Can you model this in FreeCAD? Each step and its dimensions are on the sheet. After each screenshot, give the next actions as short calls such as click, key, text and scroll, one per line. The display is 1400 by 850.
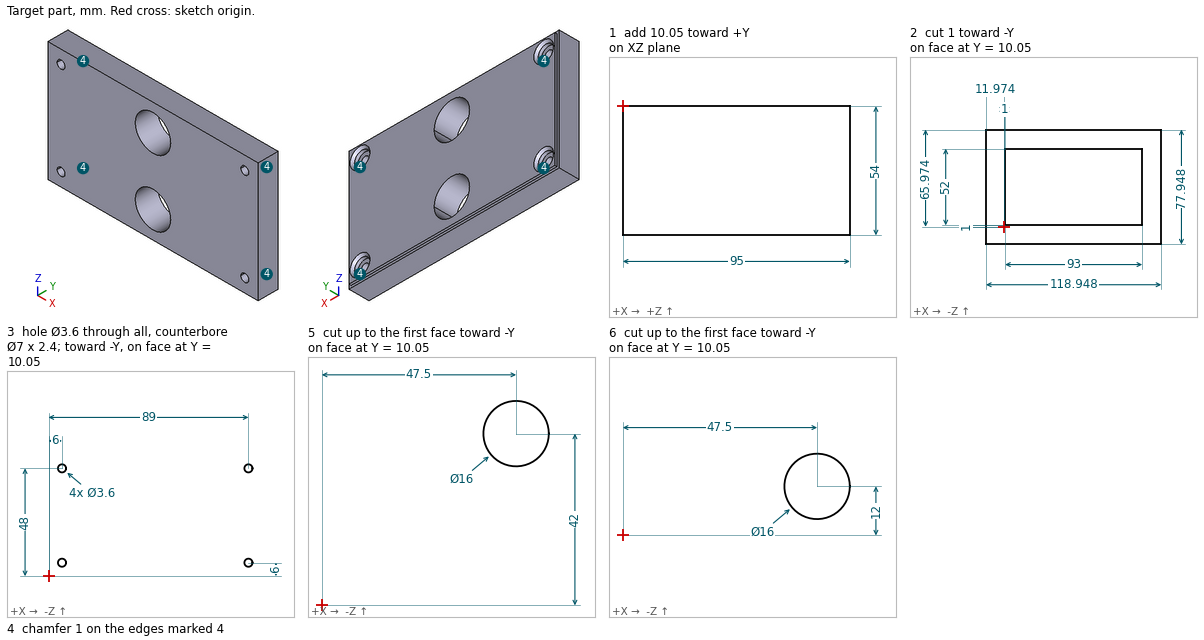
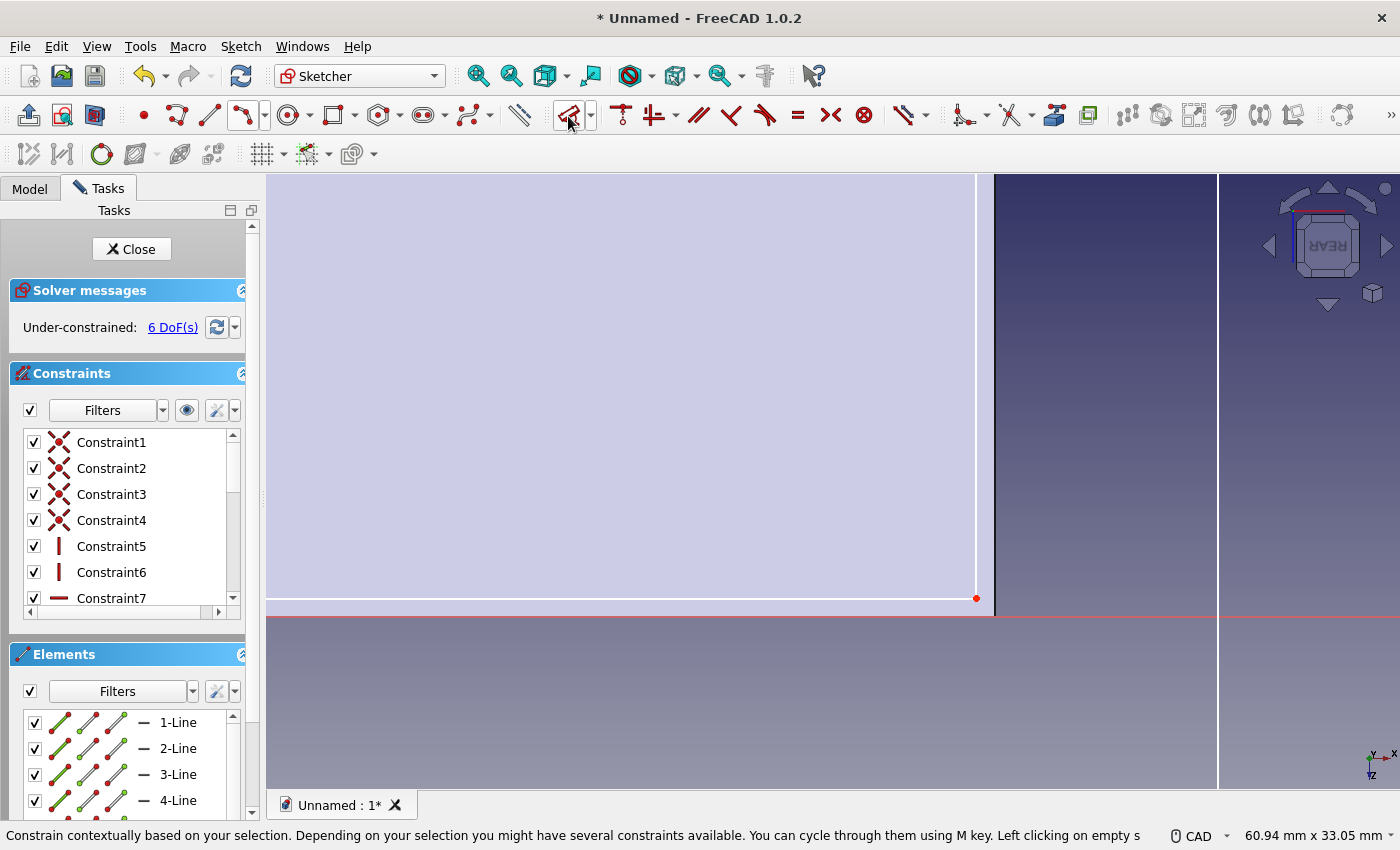
scroll(978, 602, down, 7)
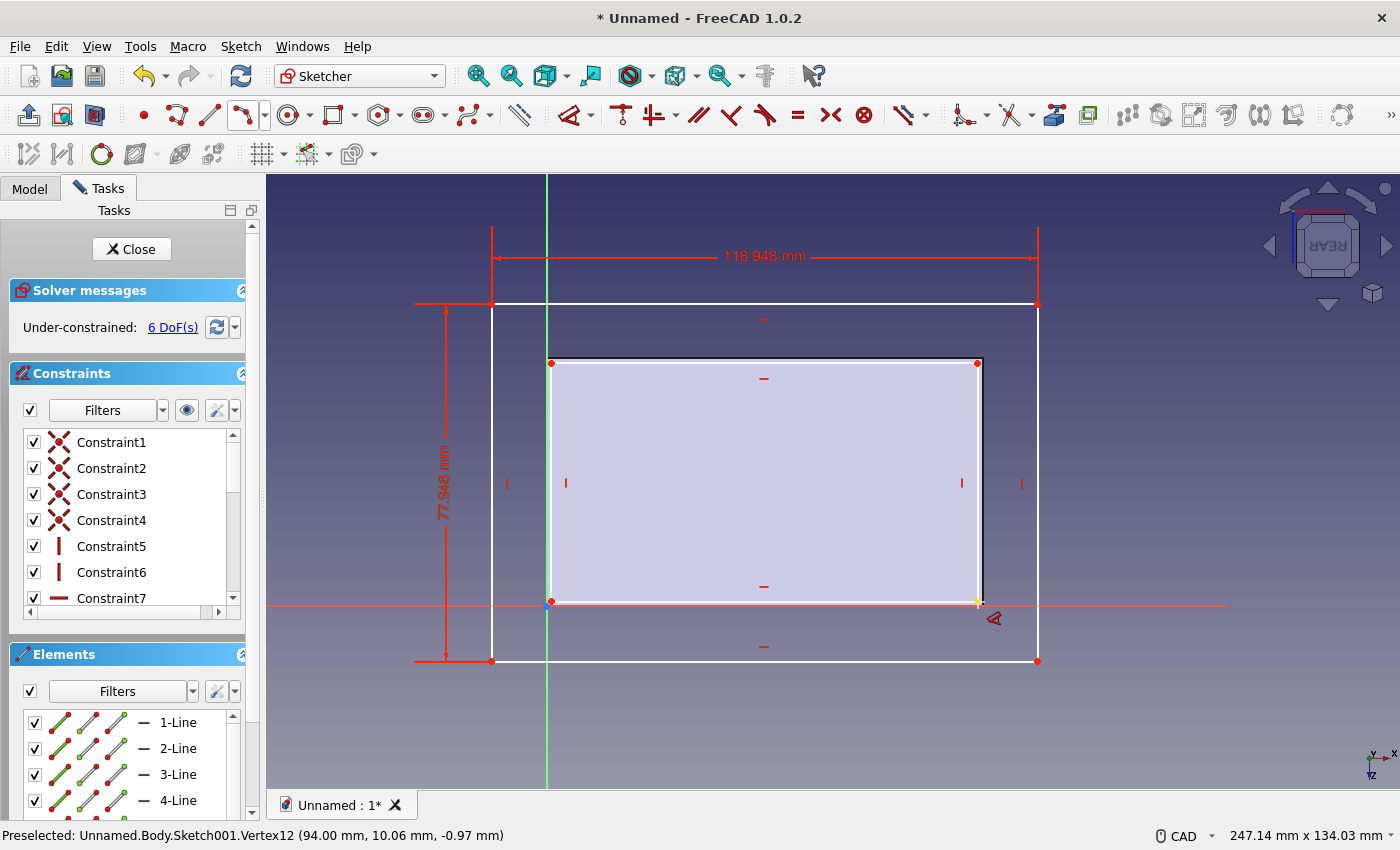
scroll(551, 435, up, 6)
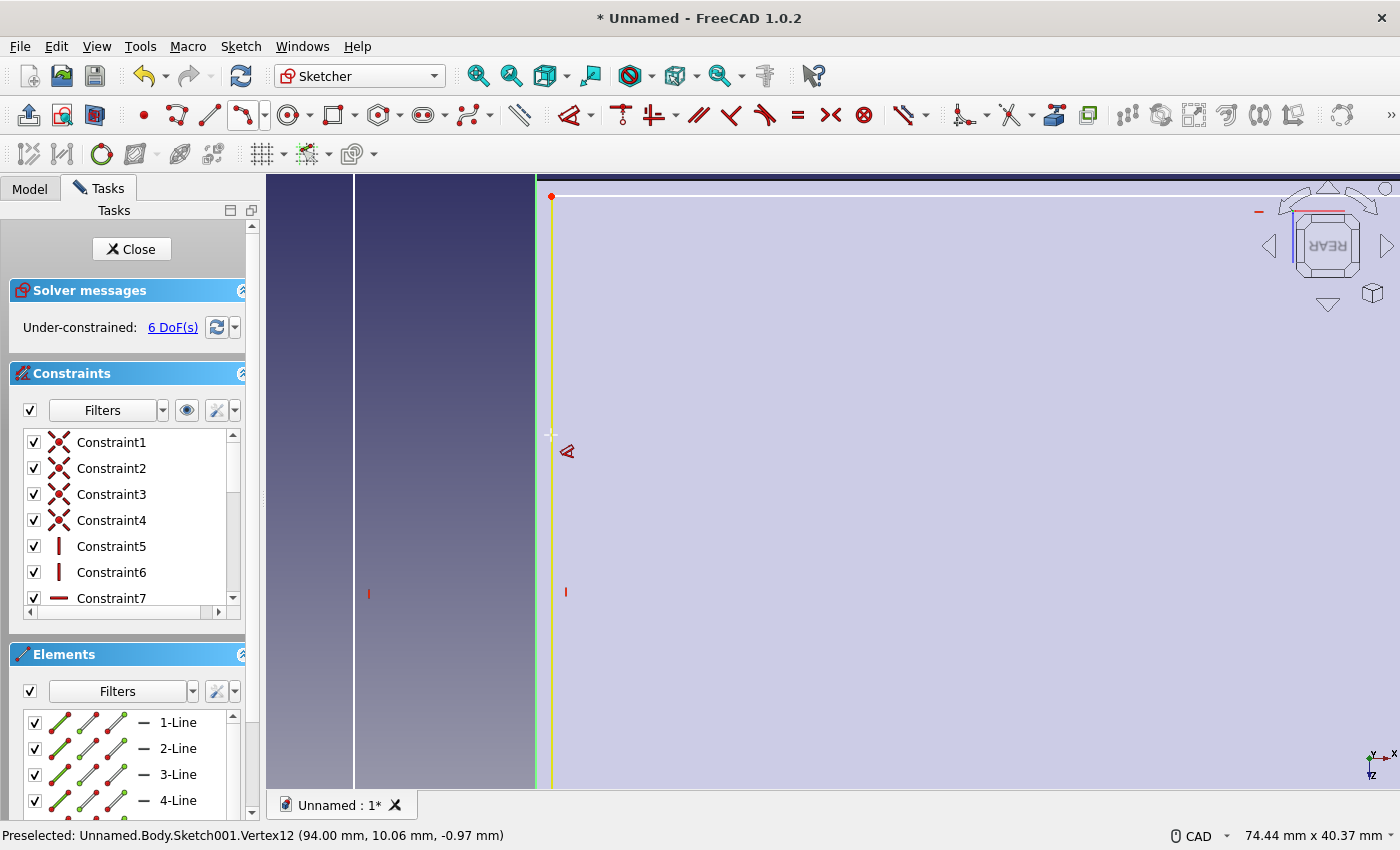
click(552, 434)
click(518, 482)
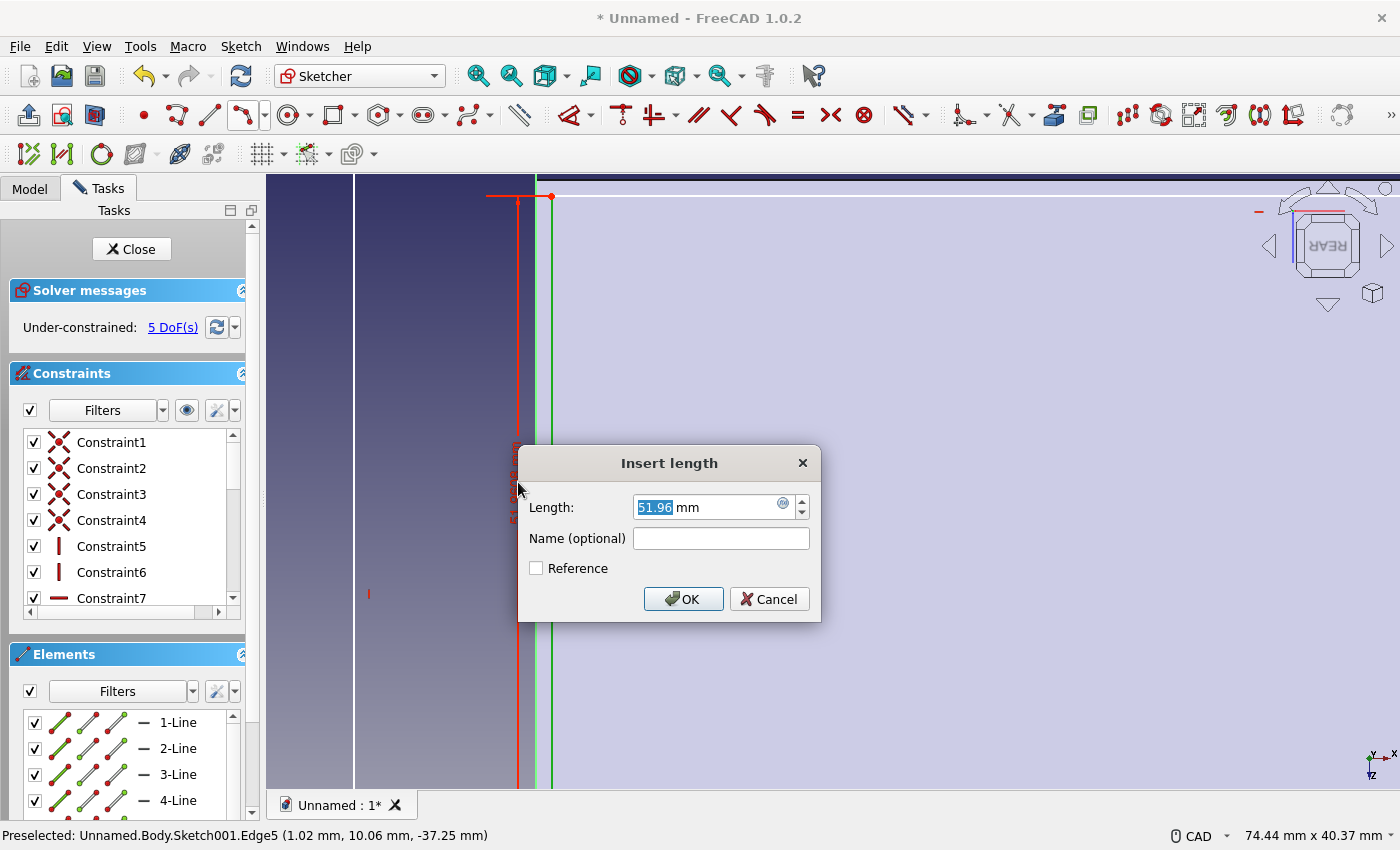
text(52)
key(Return)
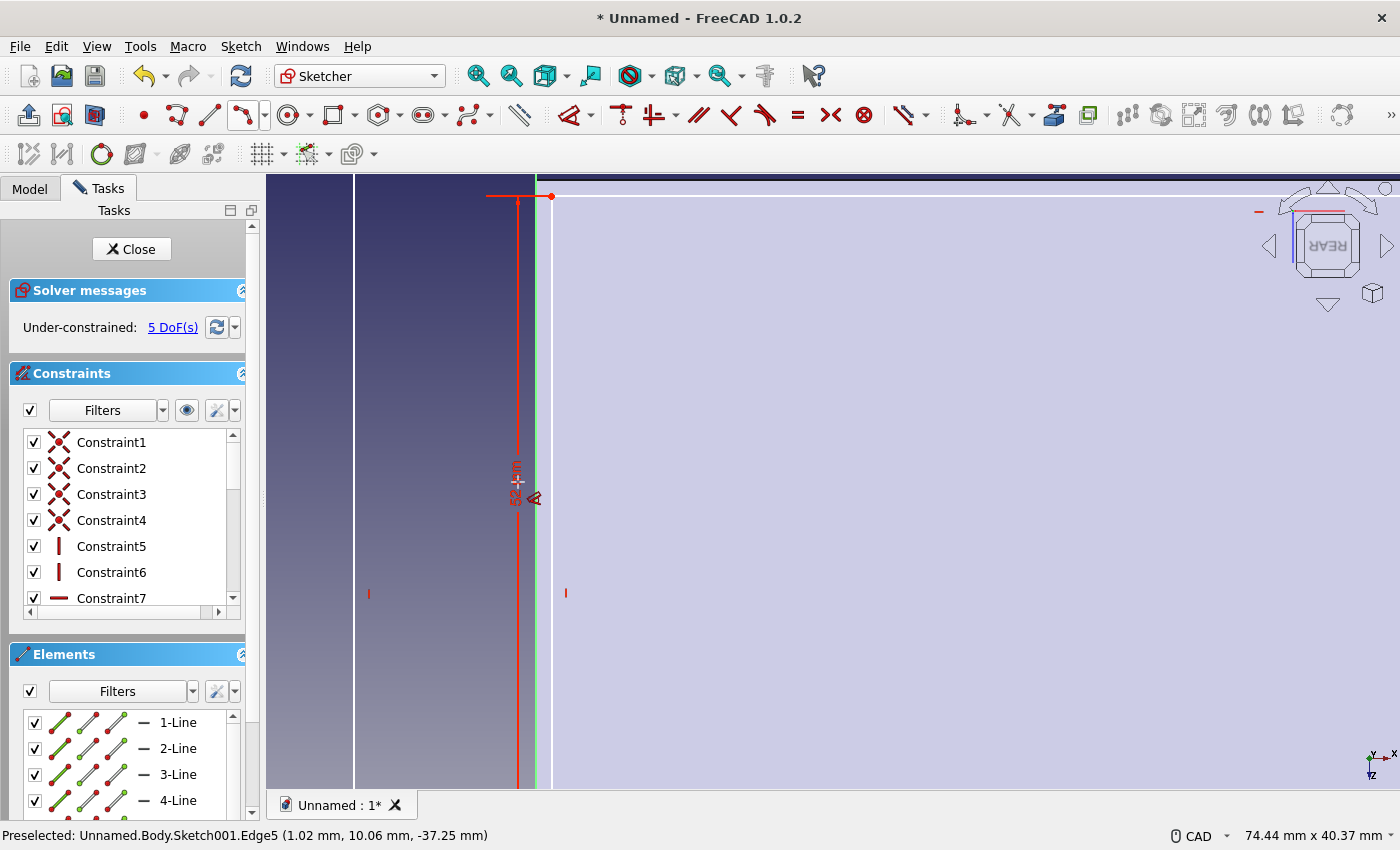
scroll(551, 434, down, 6)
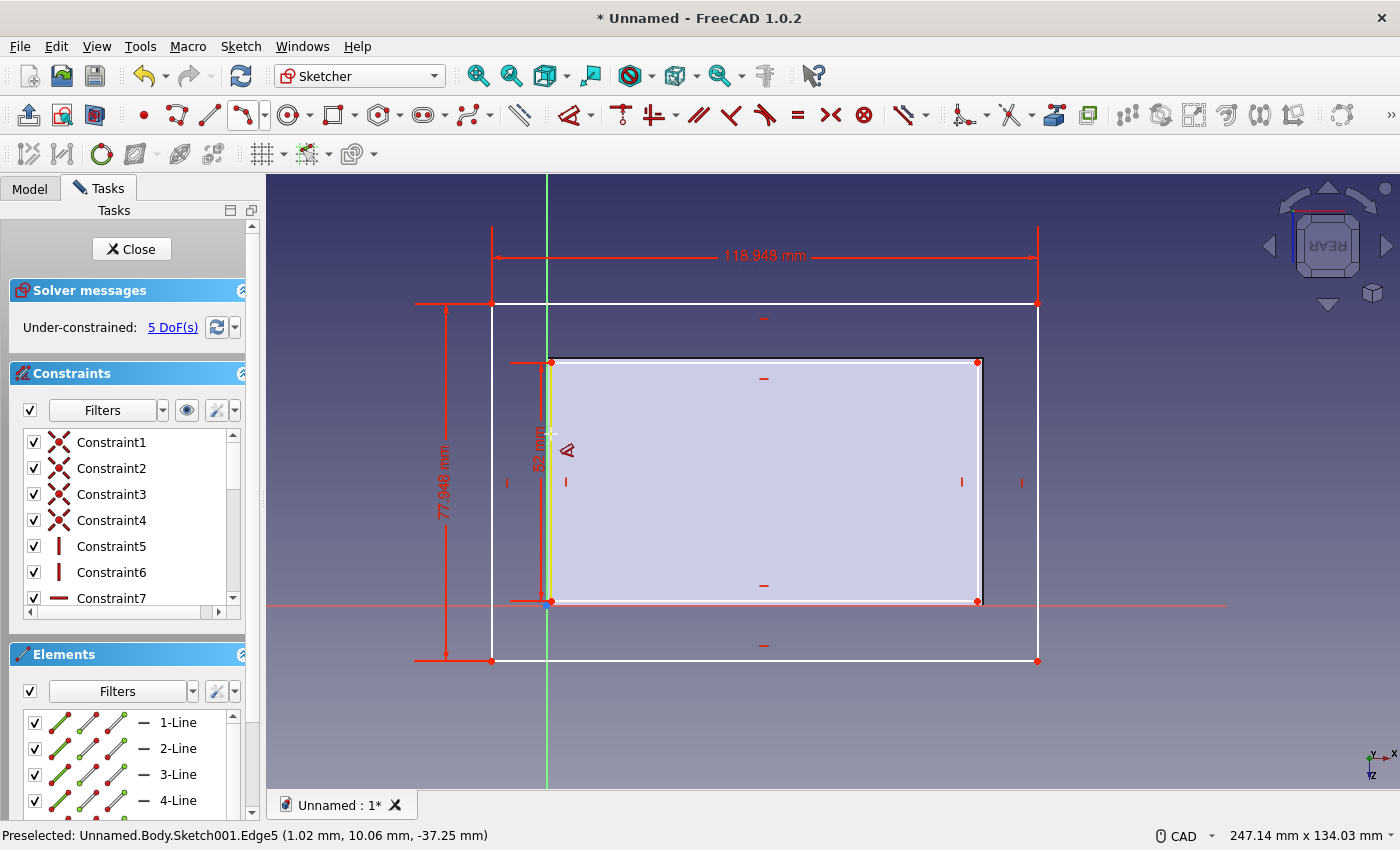
scroll(679, 601, up, 6)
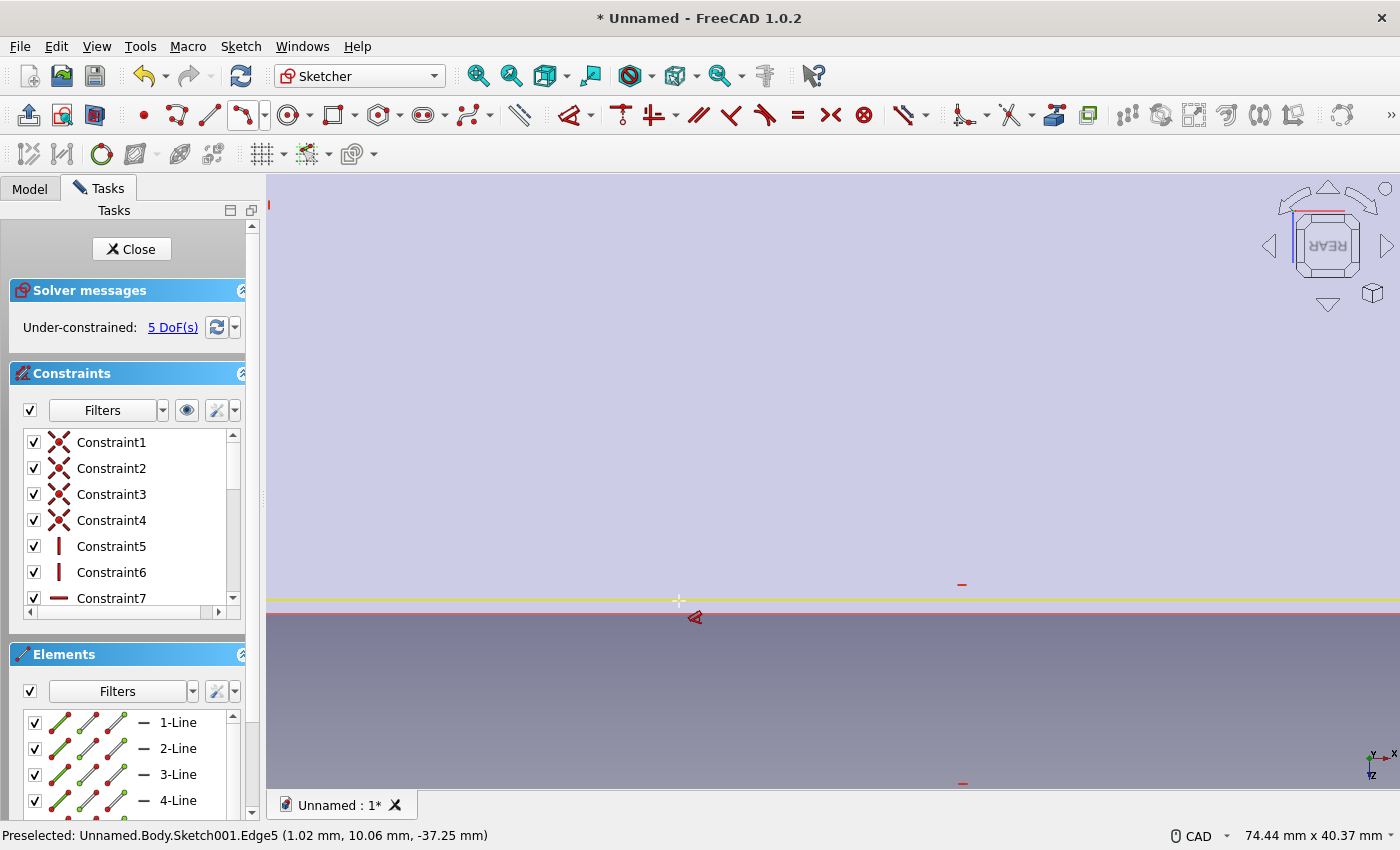
click(679, 600)
click(764, 634)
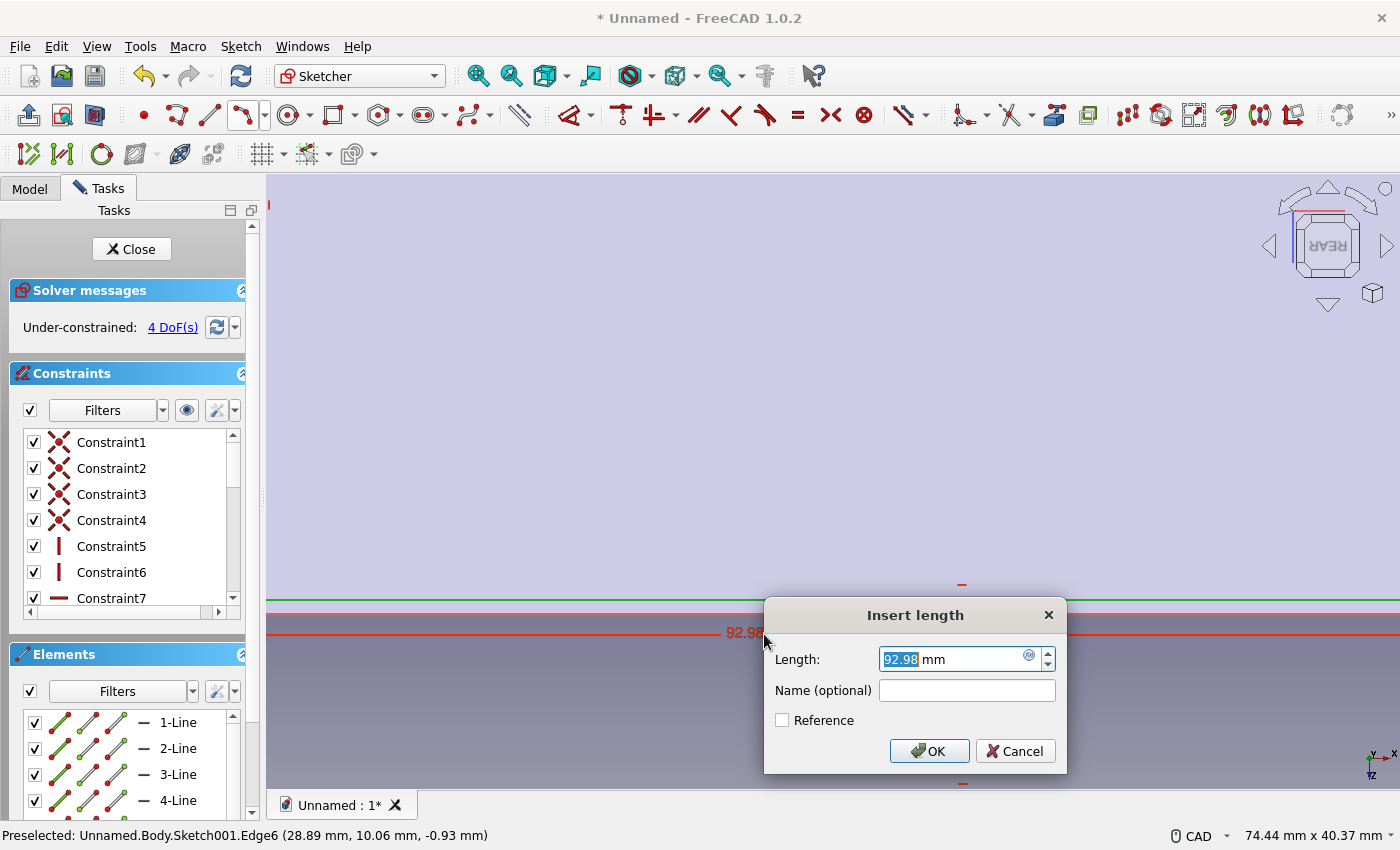
text(93)
key(Return)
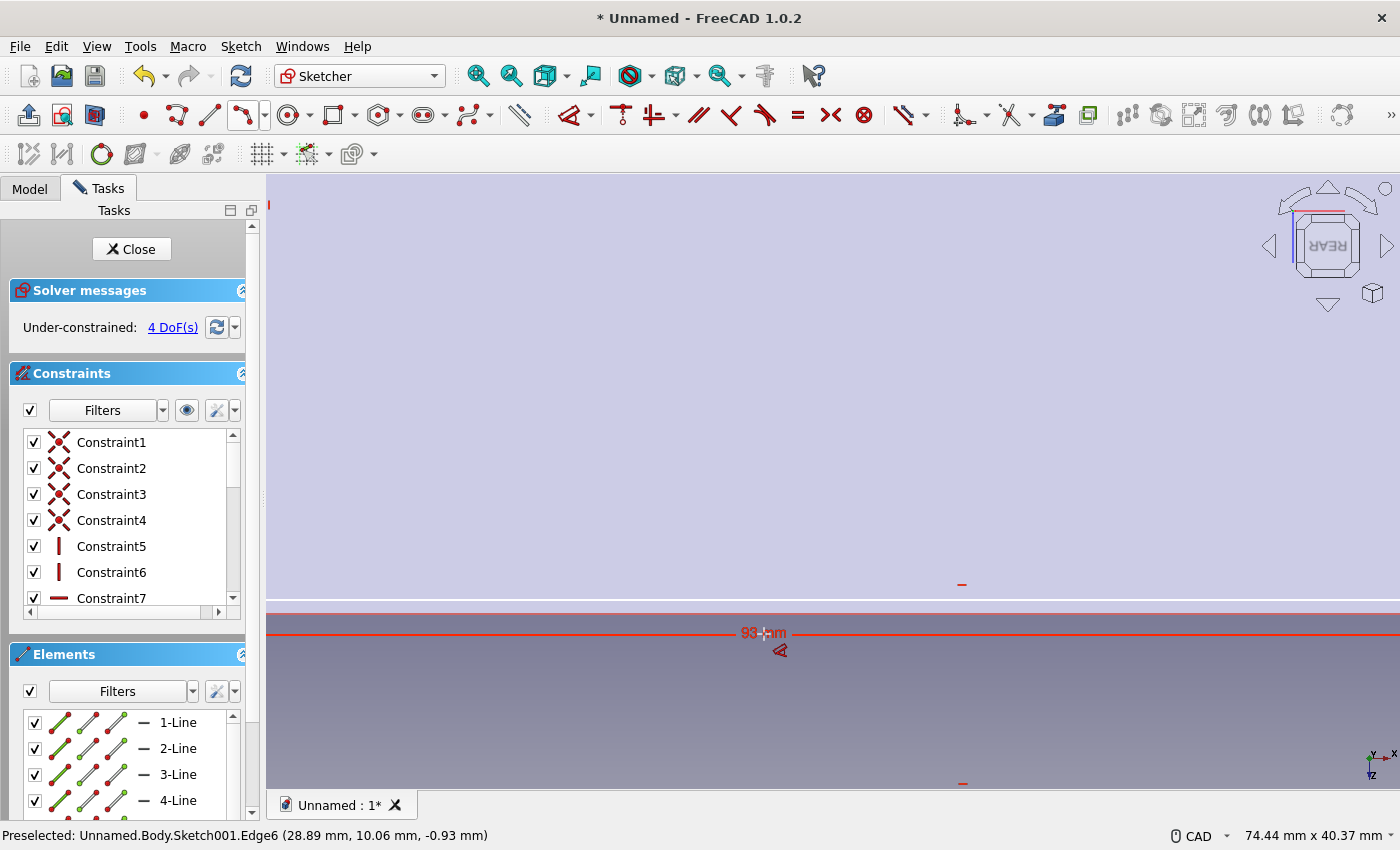
scroll(679, 601, down, 6)